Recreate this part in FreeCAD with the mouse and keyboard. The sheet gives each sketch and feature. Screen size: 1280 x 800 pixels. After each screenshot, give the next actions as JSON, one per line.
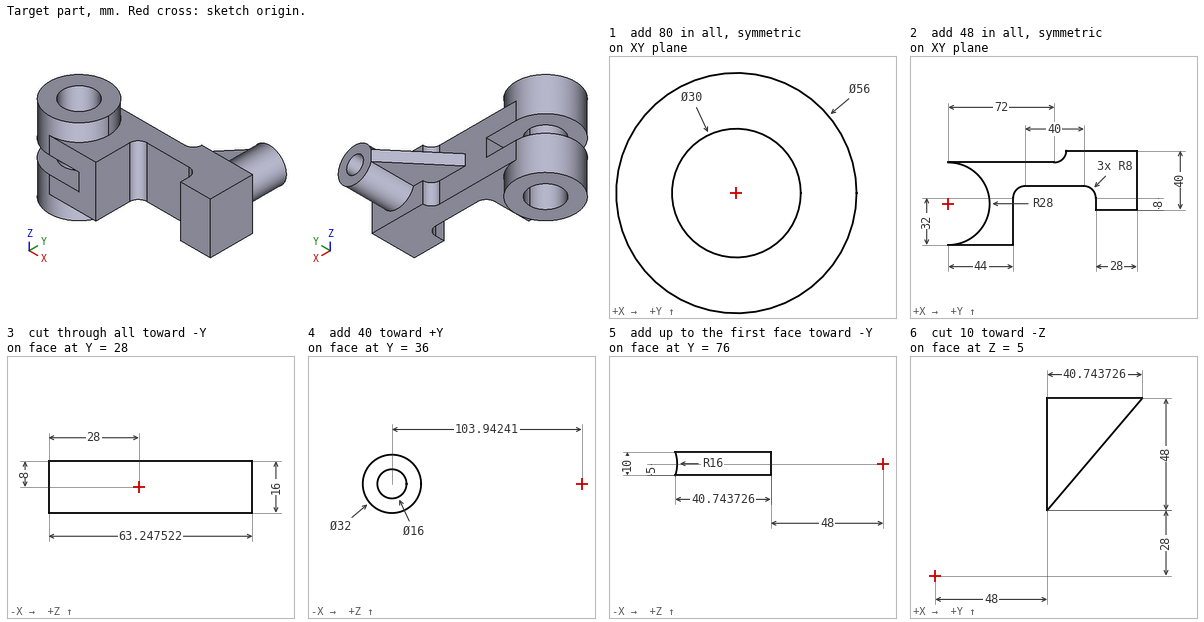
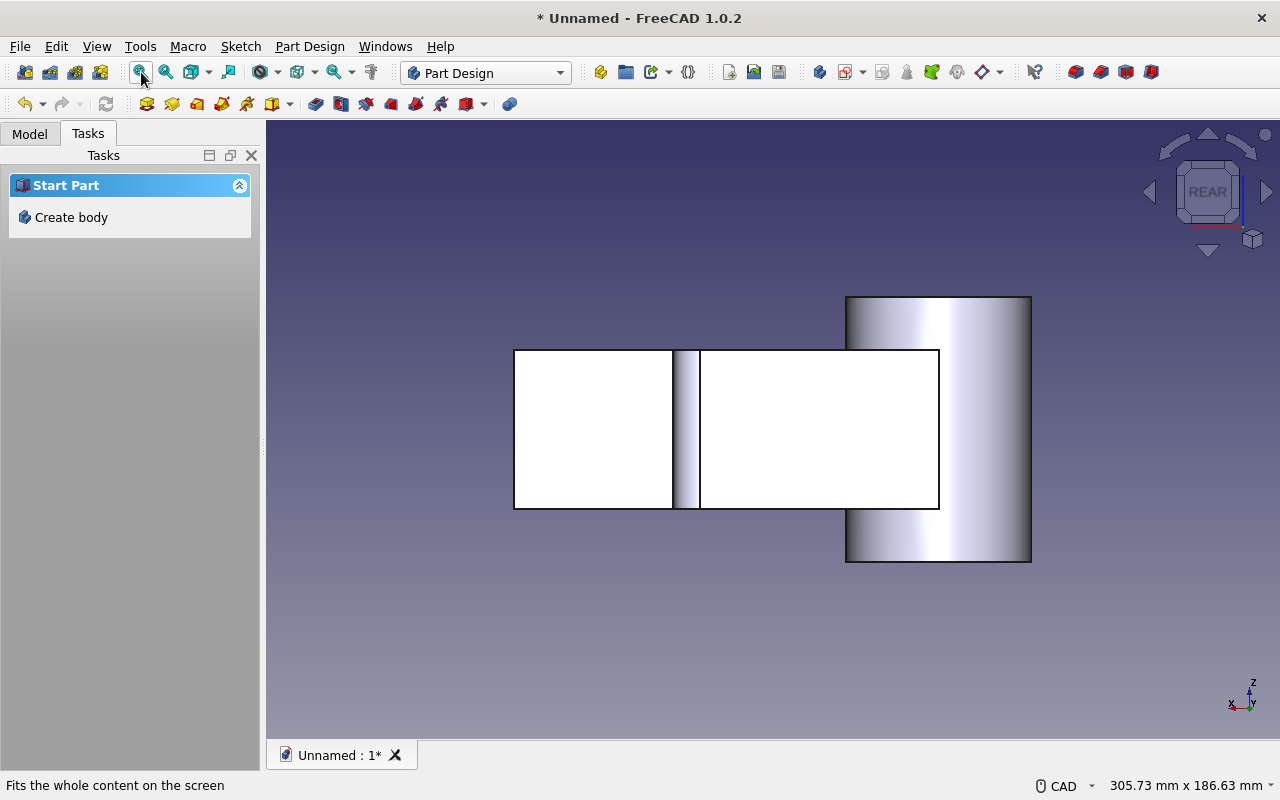
{"action": "left_click", "coordinate": [785, 428]}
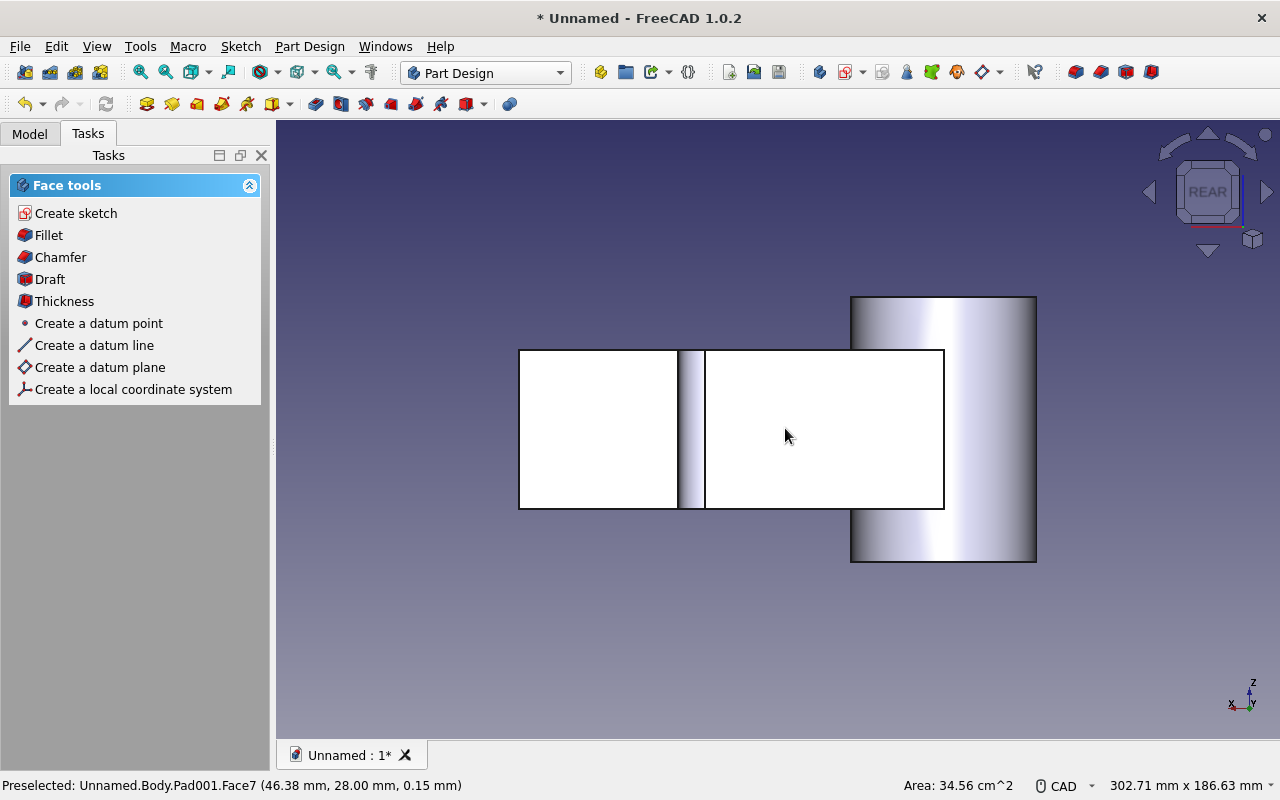
{"action": "left_click", "coordinate": [844, 72]}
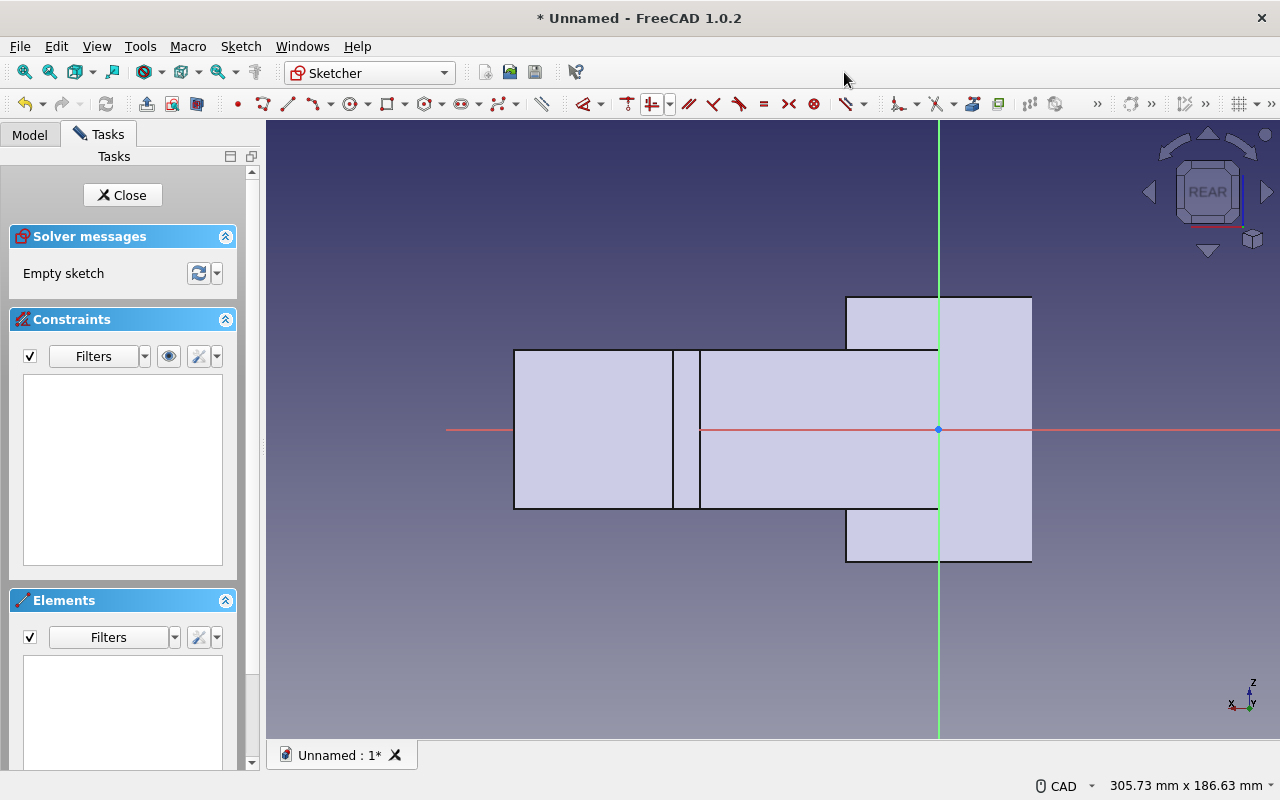
{"action": "scroll", "coordinate": [1094, 429], "scroll_direction": "up", "scroll_amount": 5}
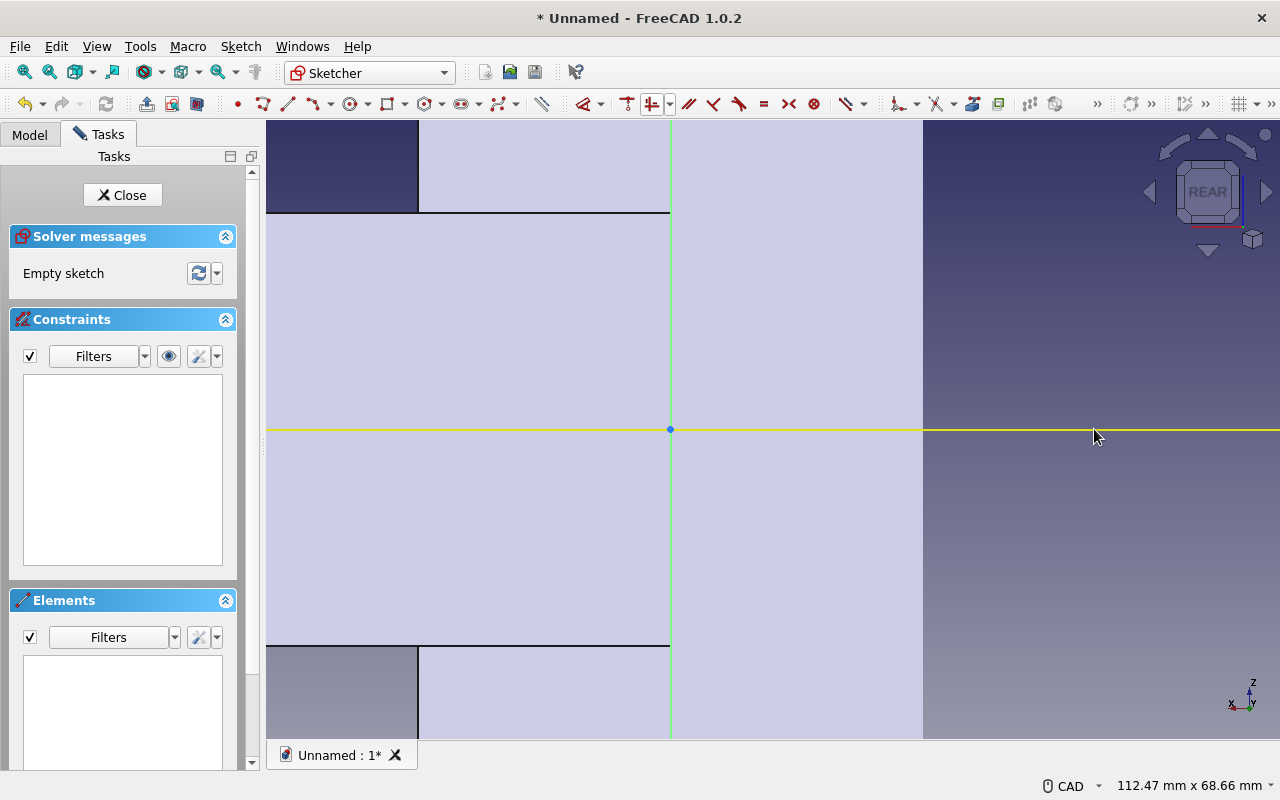
{"action": "left_click", "coordinate": [386, 104]}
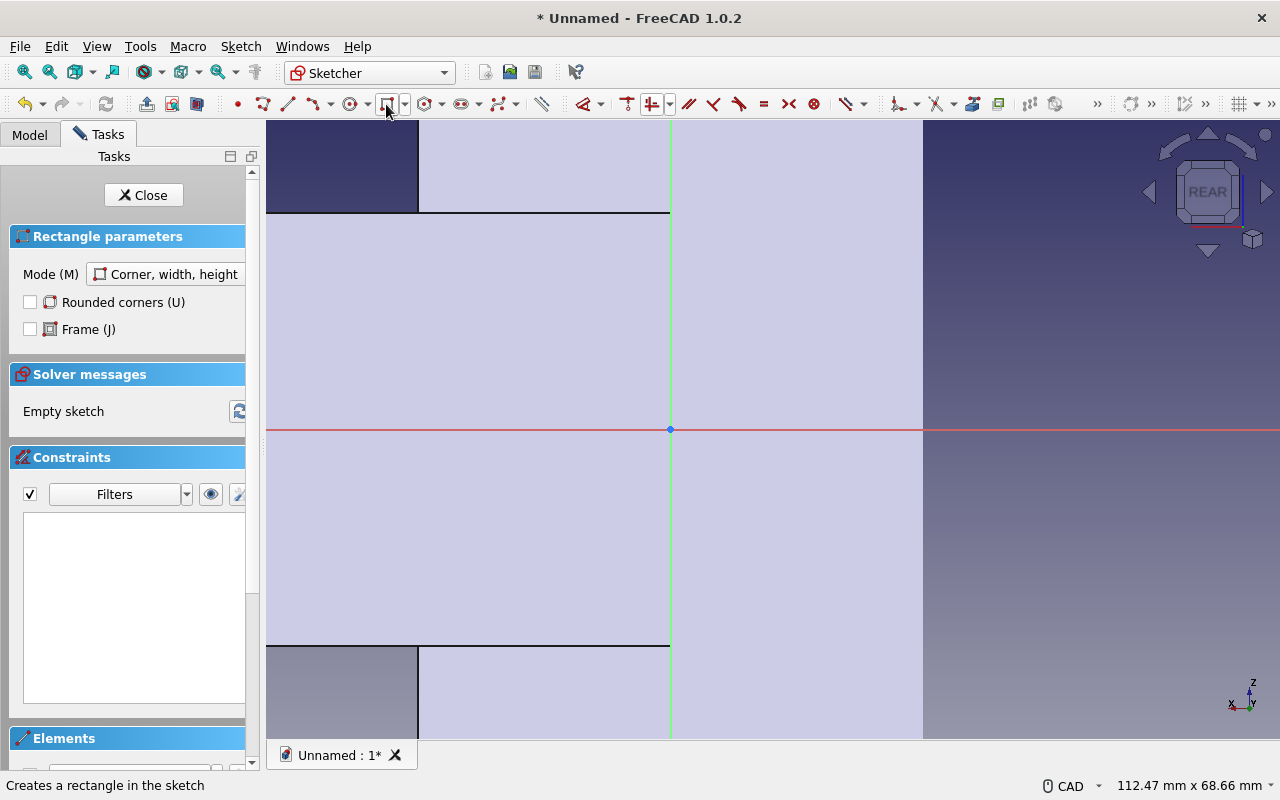
{"action": "left_click", "coordinate": [418, 357]}
{"action": "mouse_move", "coordinate": [989, 502]}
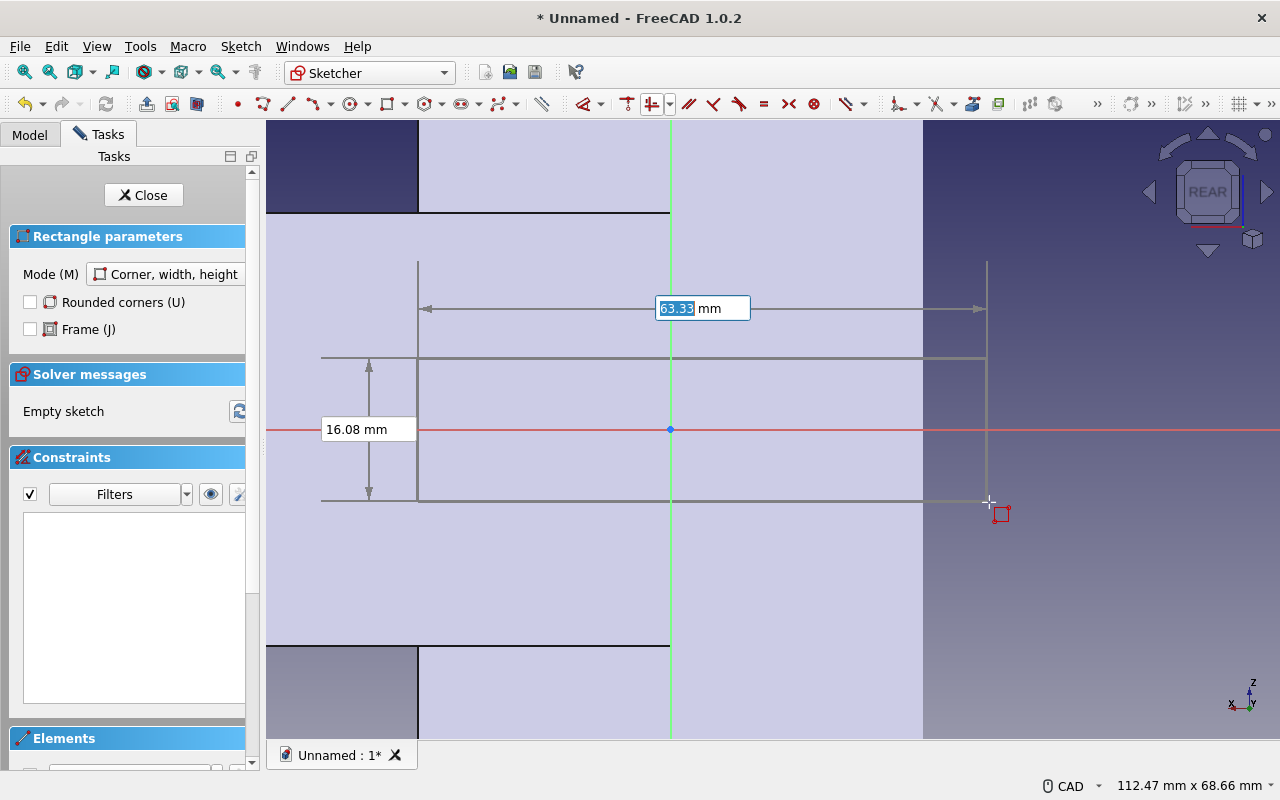
{"action": "type", "text": "63.247522"}
{"action": "key", "text": "Tab"}
{"action": "type", "text": "16"}
{"action": "key", "text": "Return"}
{"action": "key", "text": "Escape"}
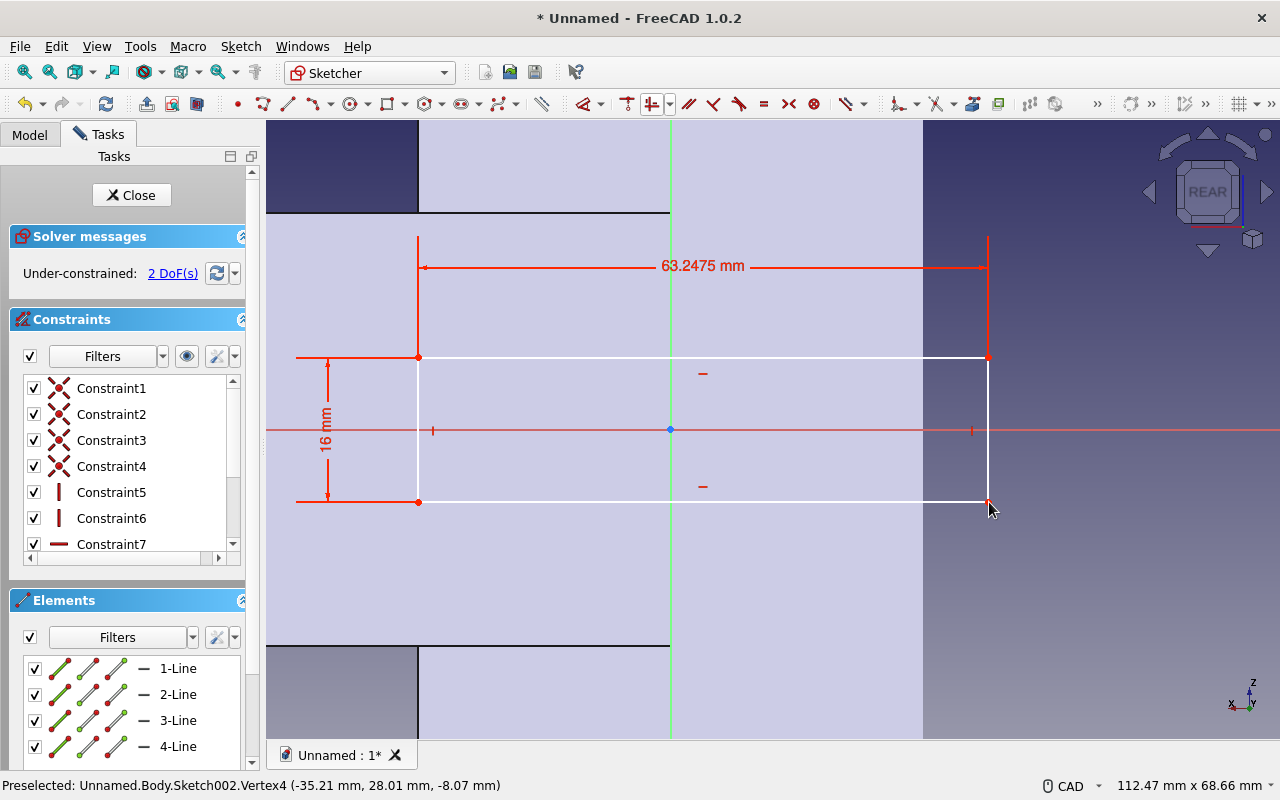
{"action": "left_click", "coordinate": [582, 104]}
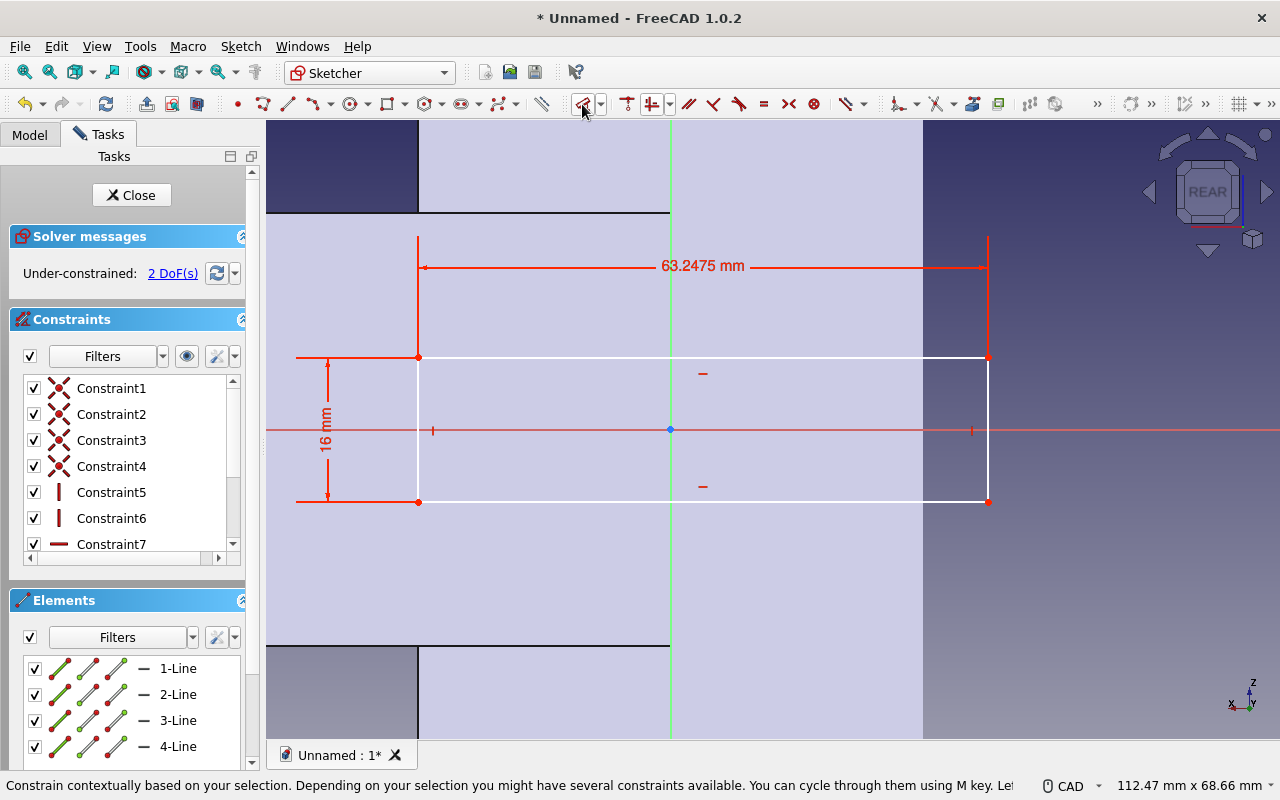
{"action": "left_click", "coordinate": [418, 358]}
{"action": "left_click", "coordinate": [384, 394]}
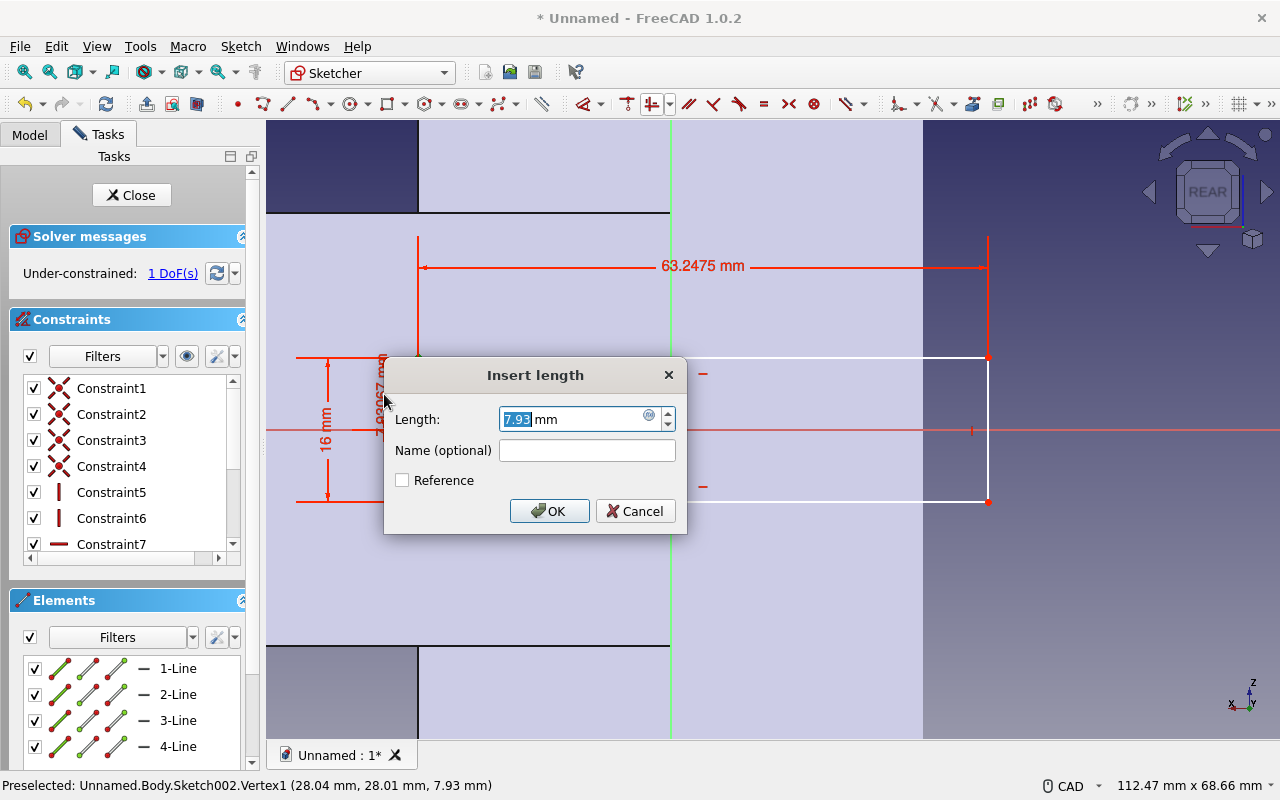
{"action": "type", "text": "8"}
{"action": "key", "text": "Return"}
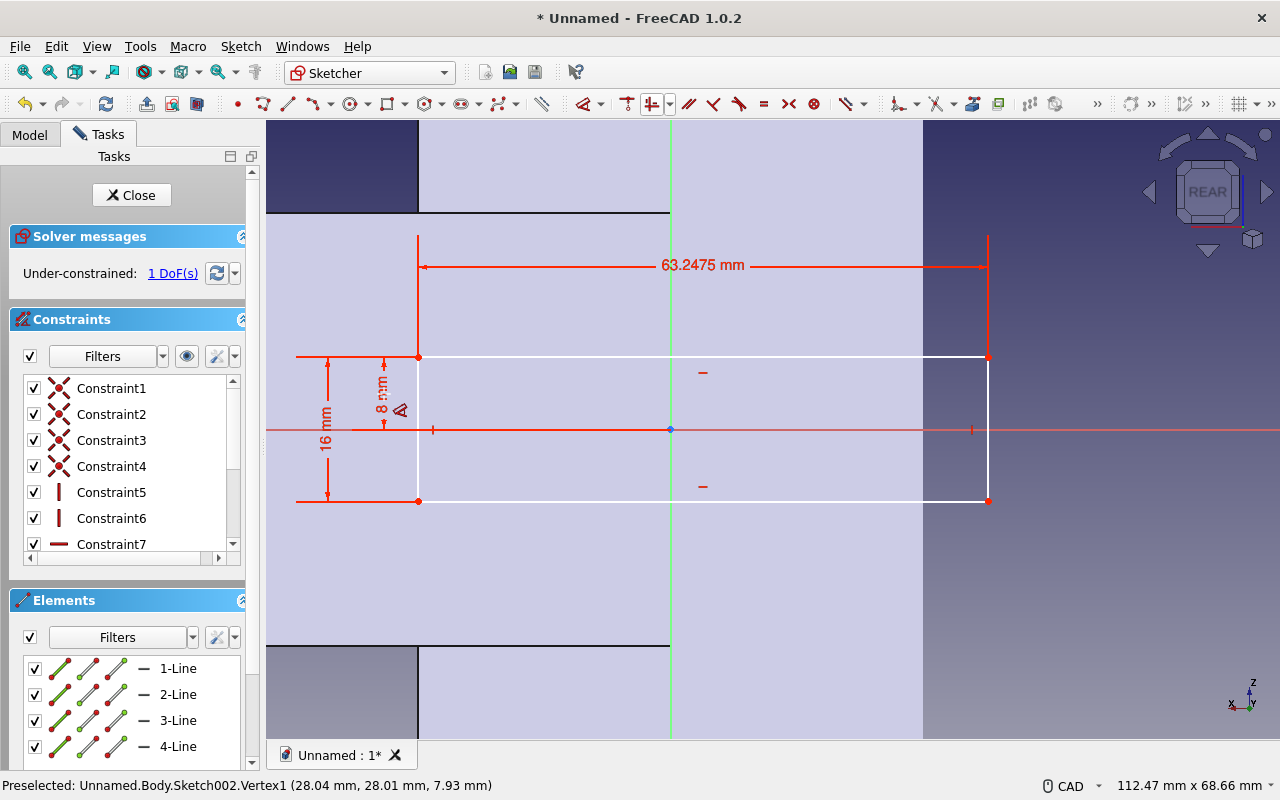
{"action": "left_click", "coordinate": [418, 357]}
{"action": "left_click", "coordinate": [544, 323]}